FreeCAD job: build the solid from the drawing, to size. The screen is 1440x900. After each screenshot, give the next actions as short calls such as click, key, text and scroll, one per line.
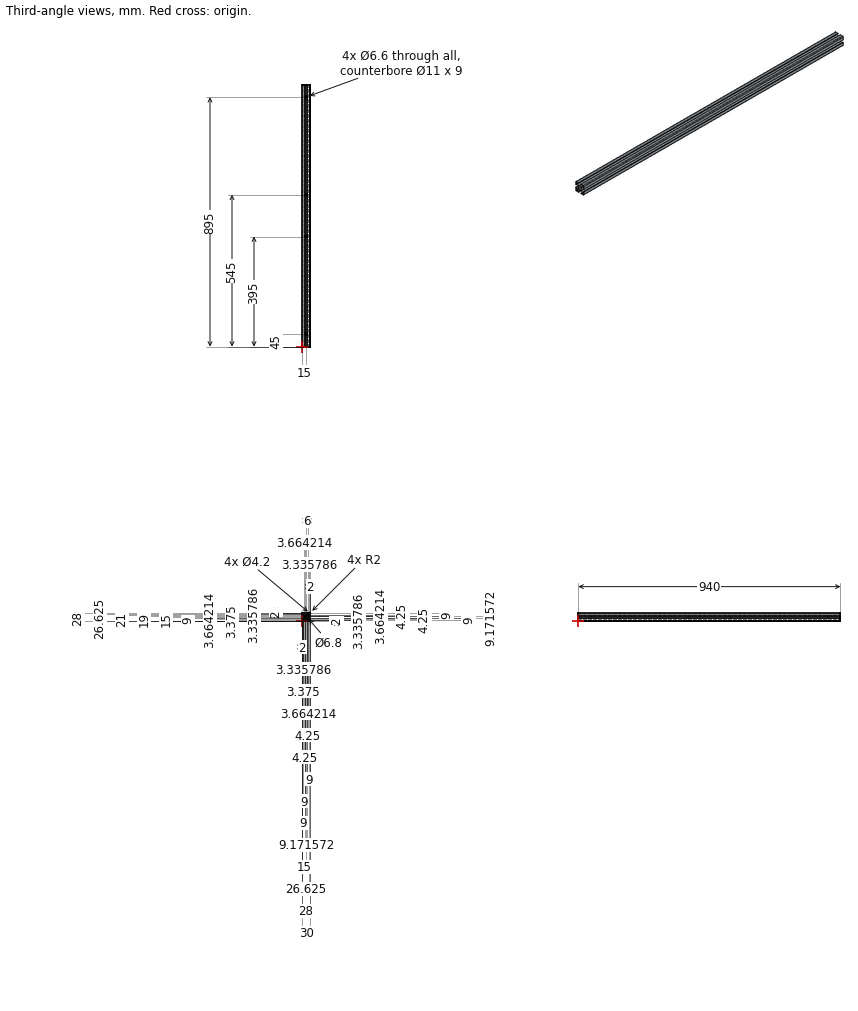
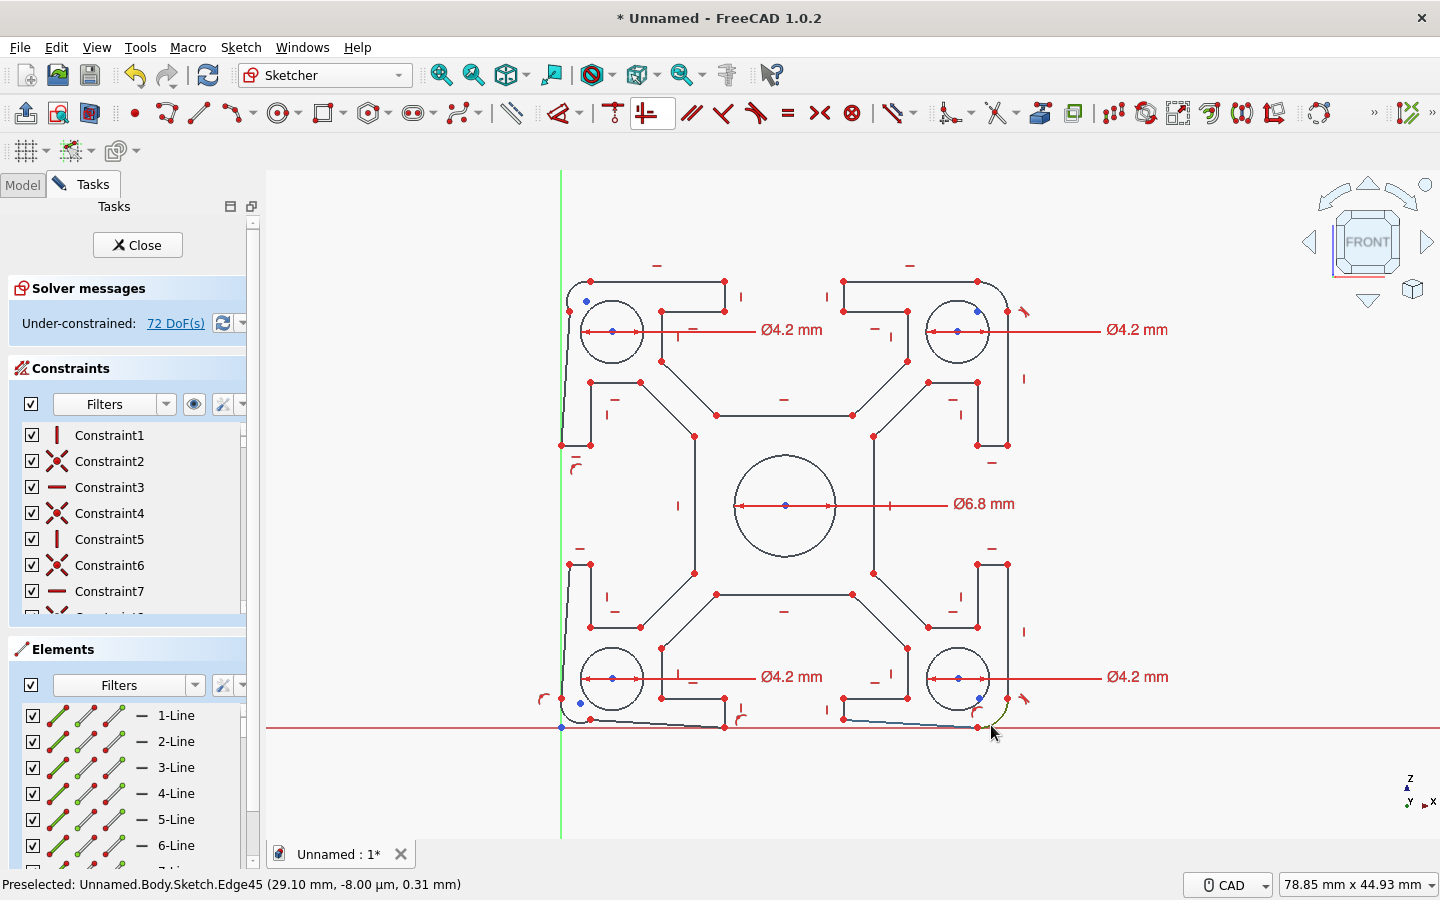
click(756, 114)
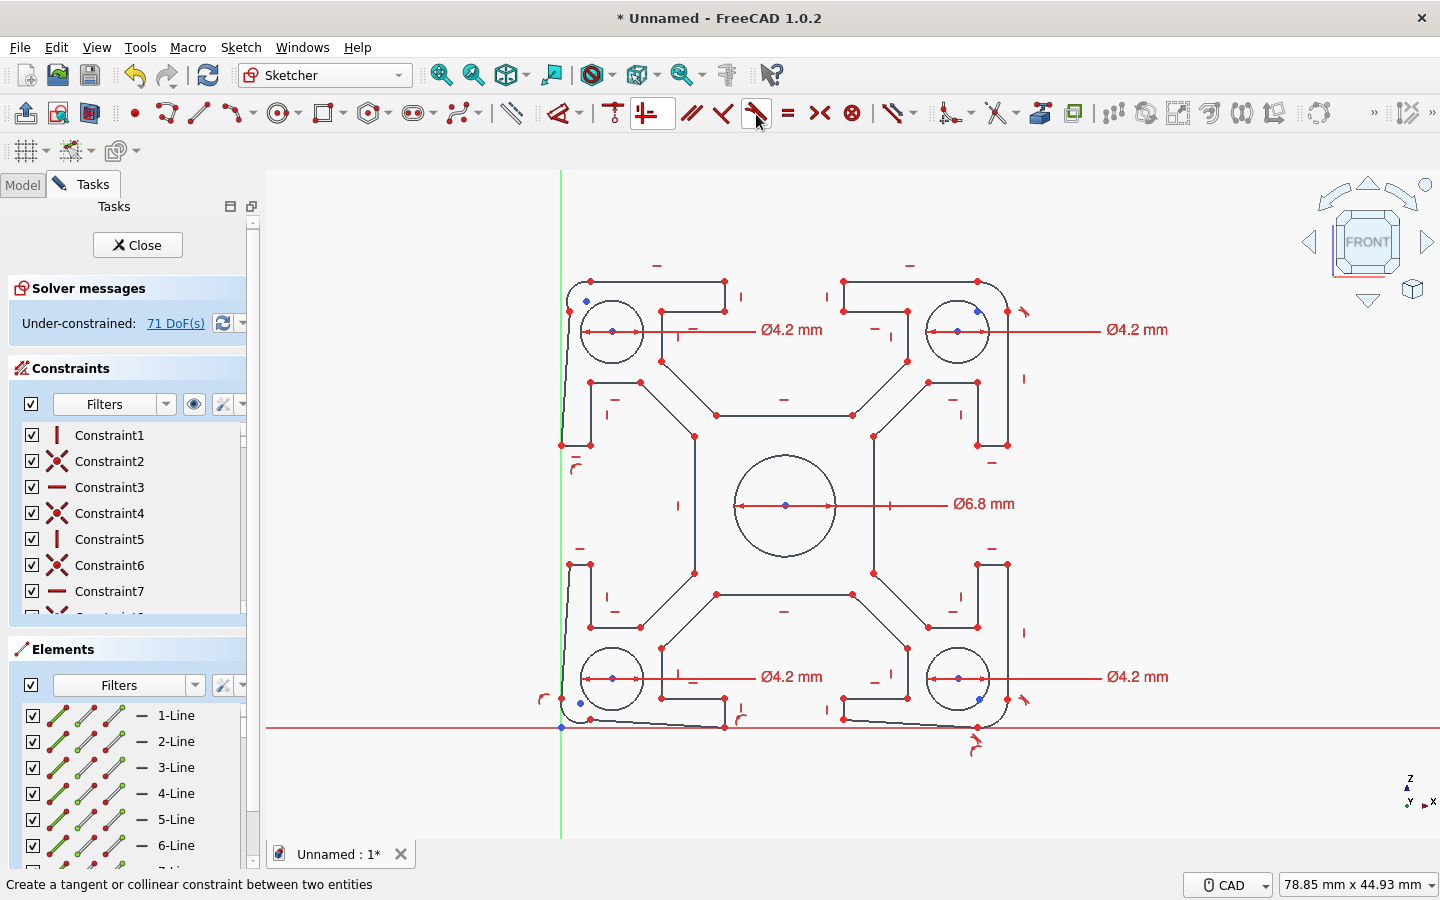
click(685, 726)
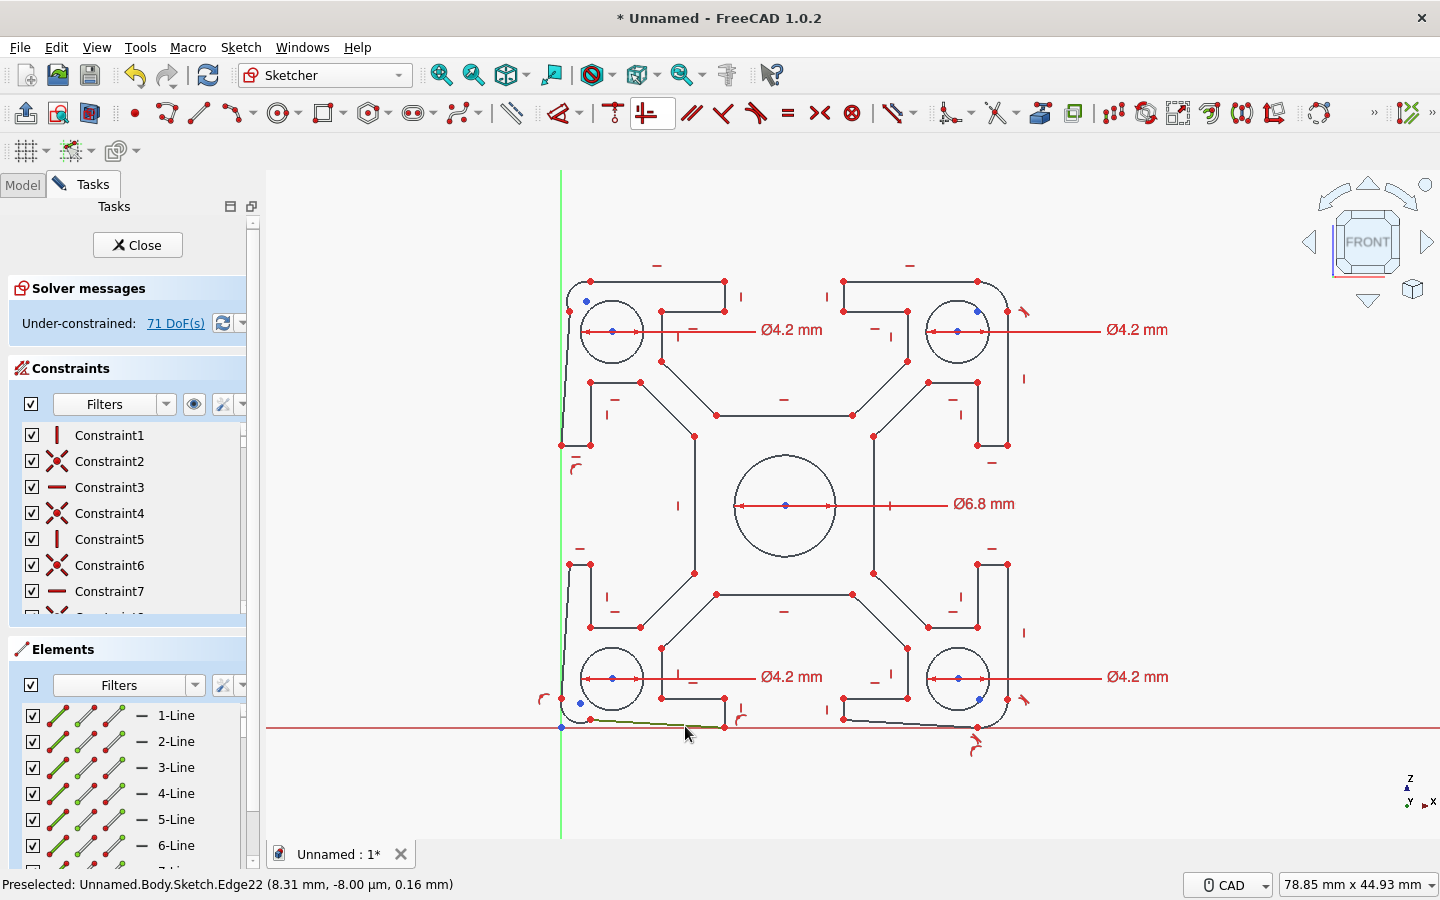
click(563, 712)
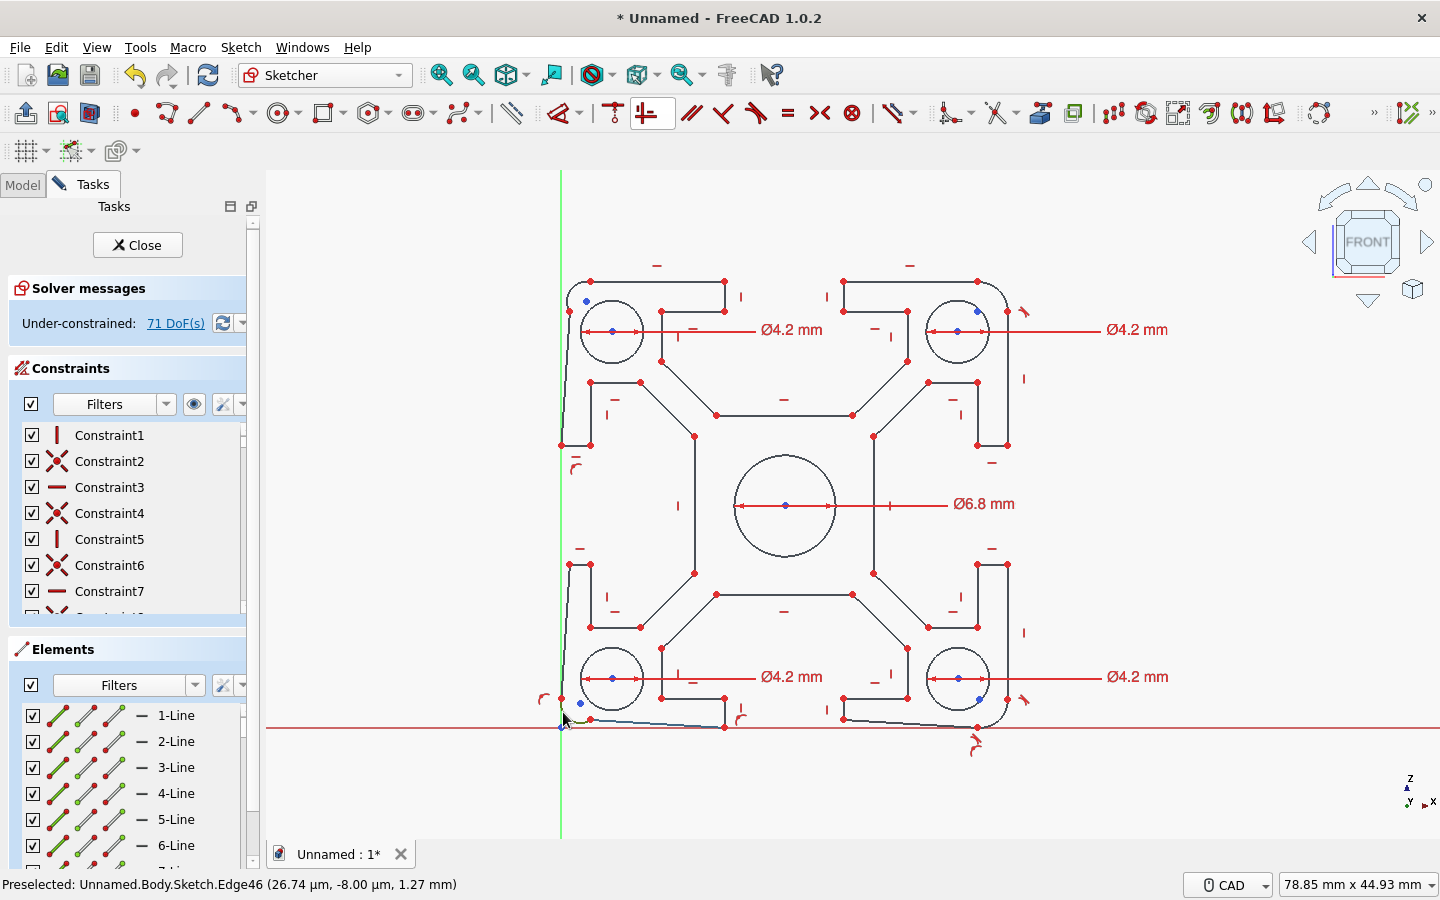
click(756, 114)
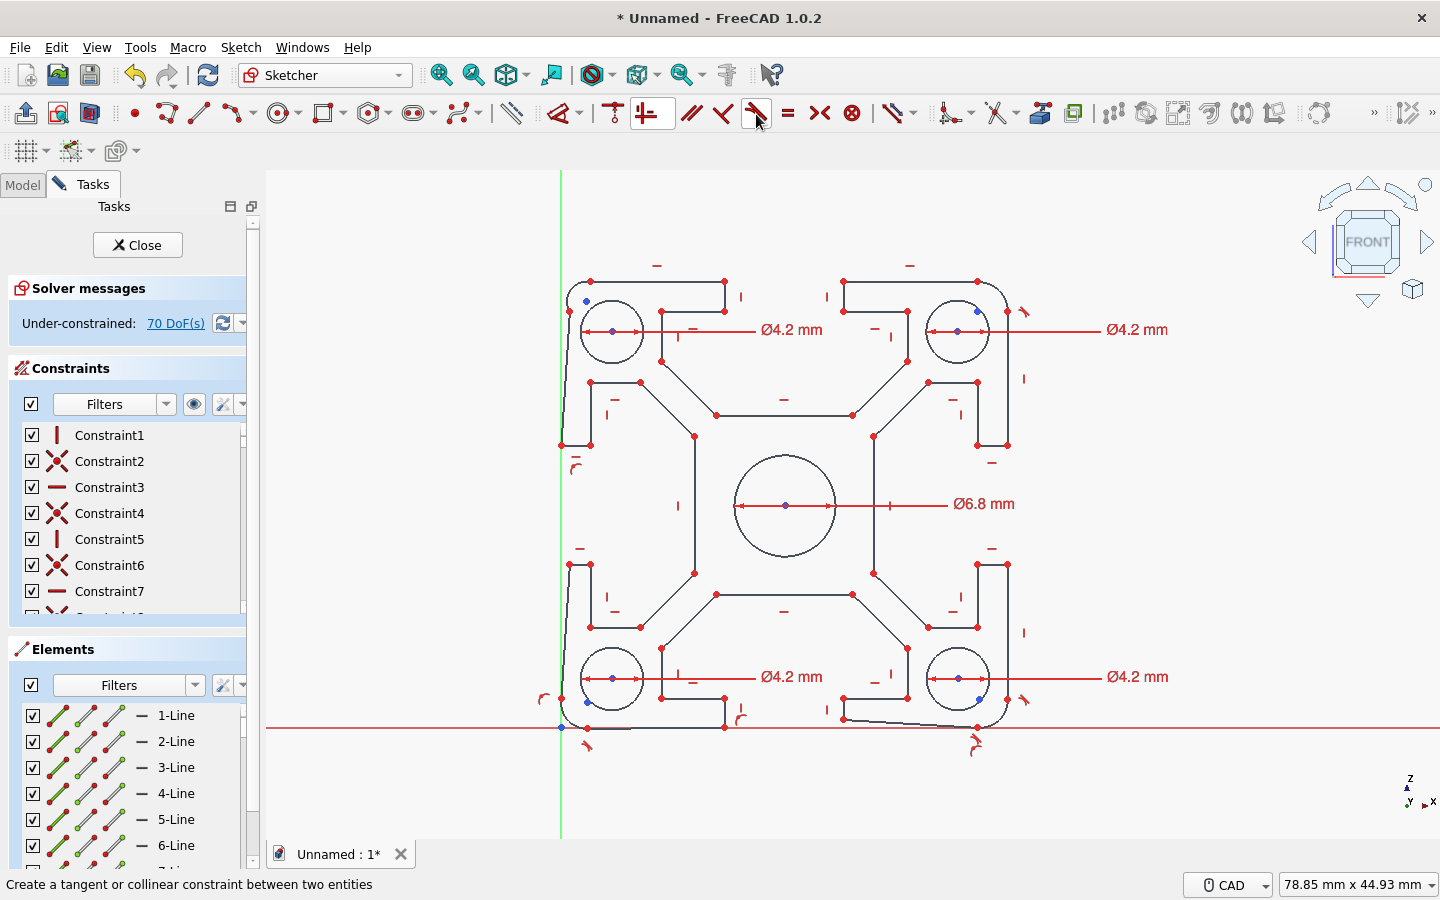
click(564, 659)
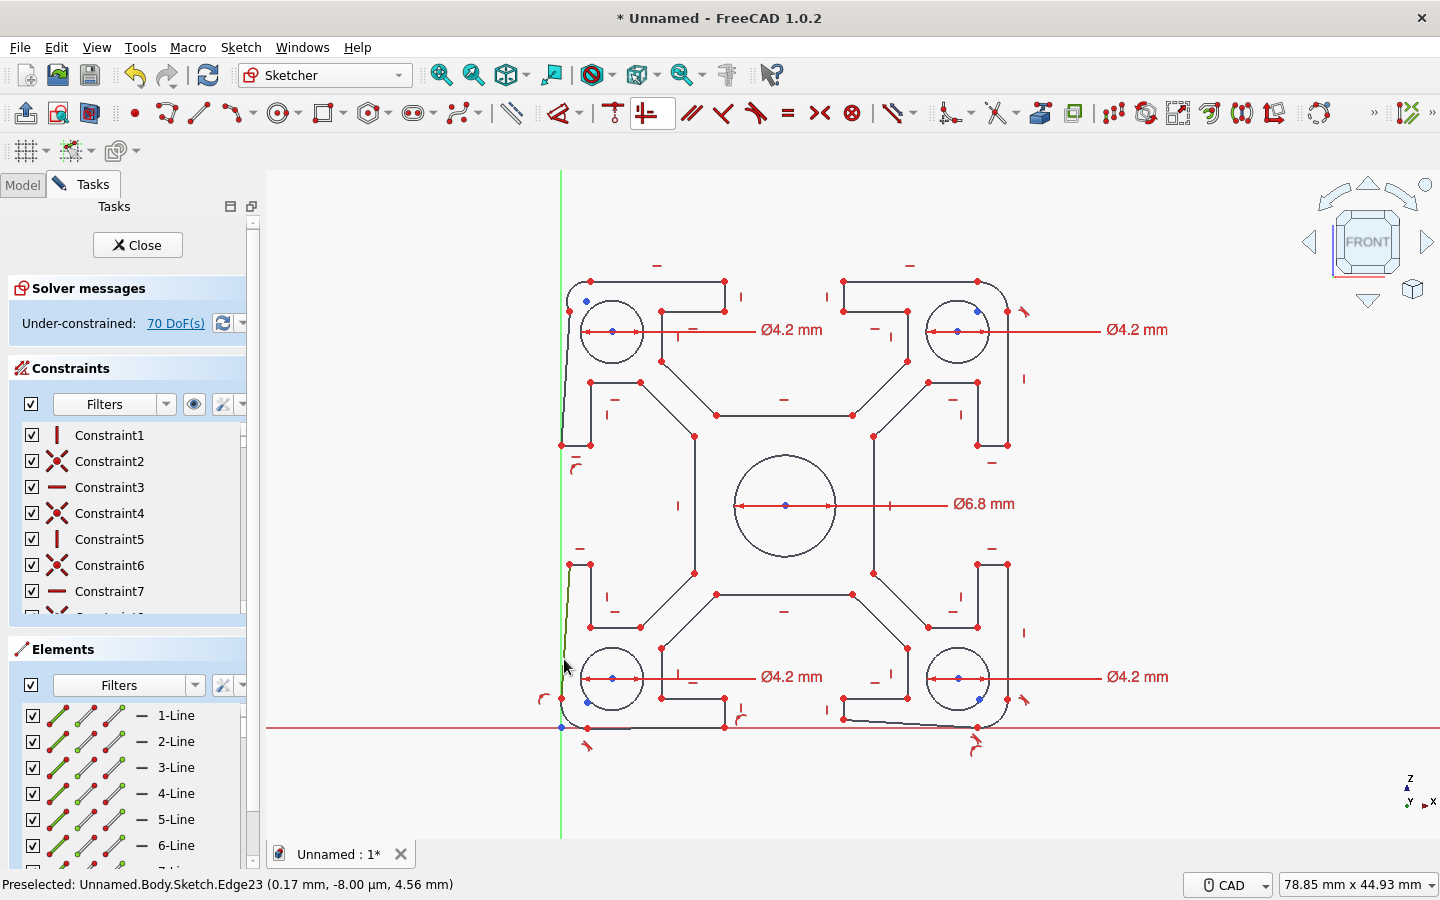
click(563, 712)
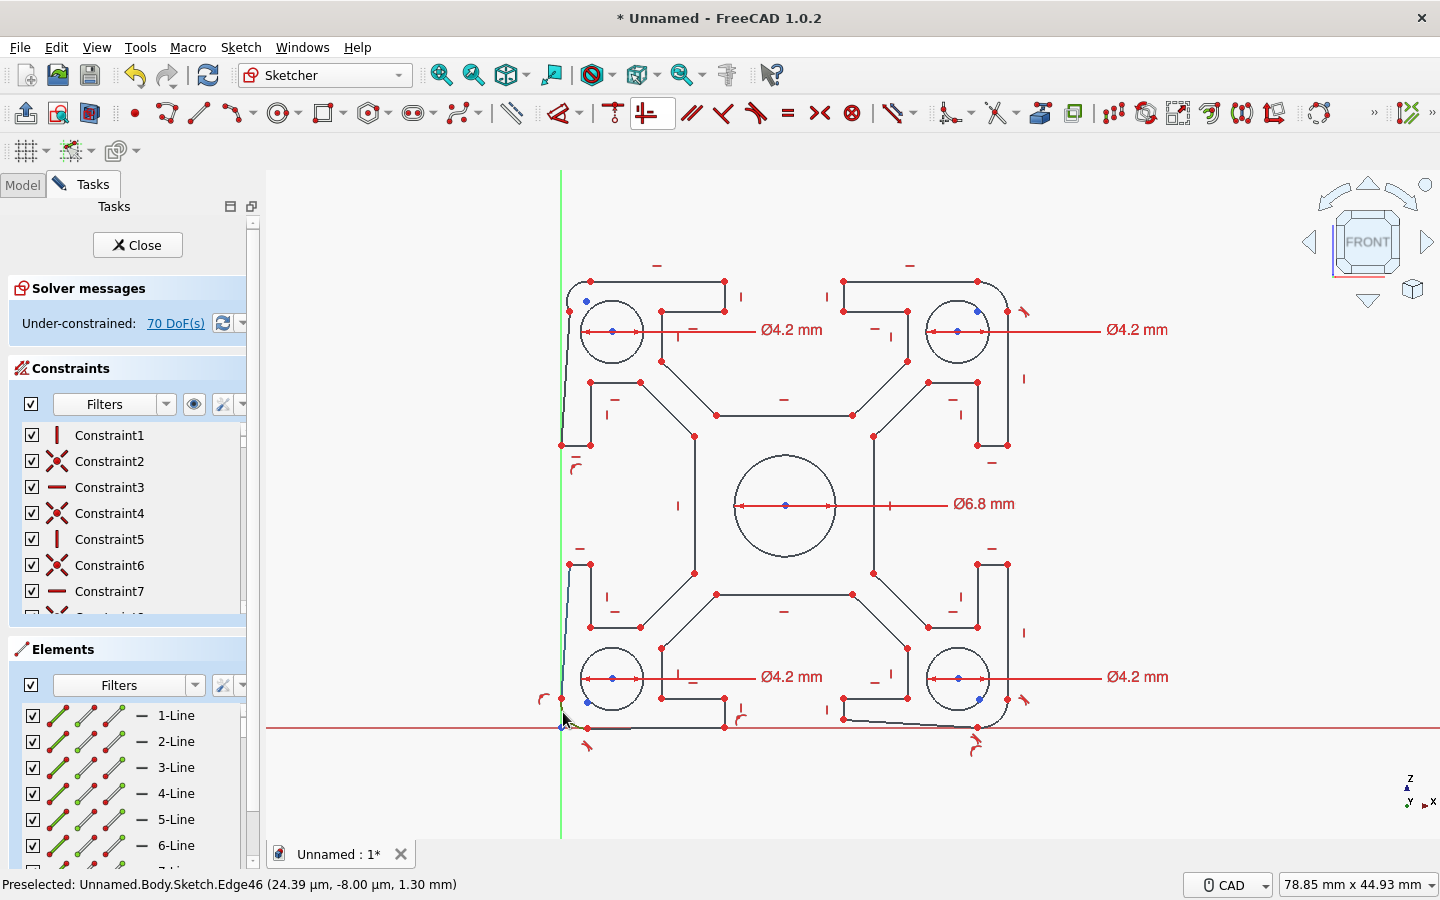
click(756, 114)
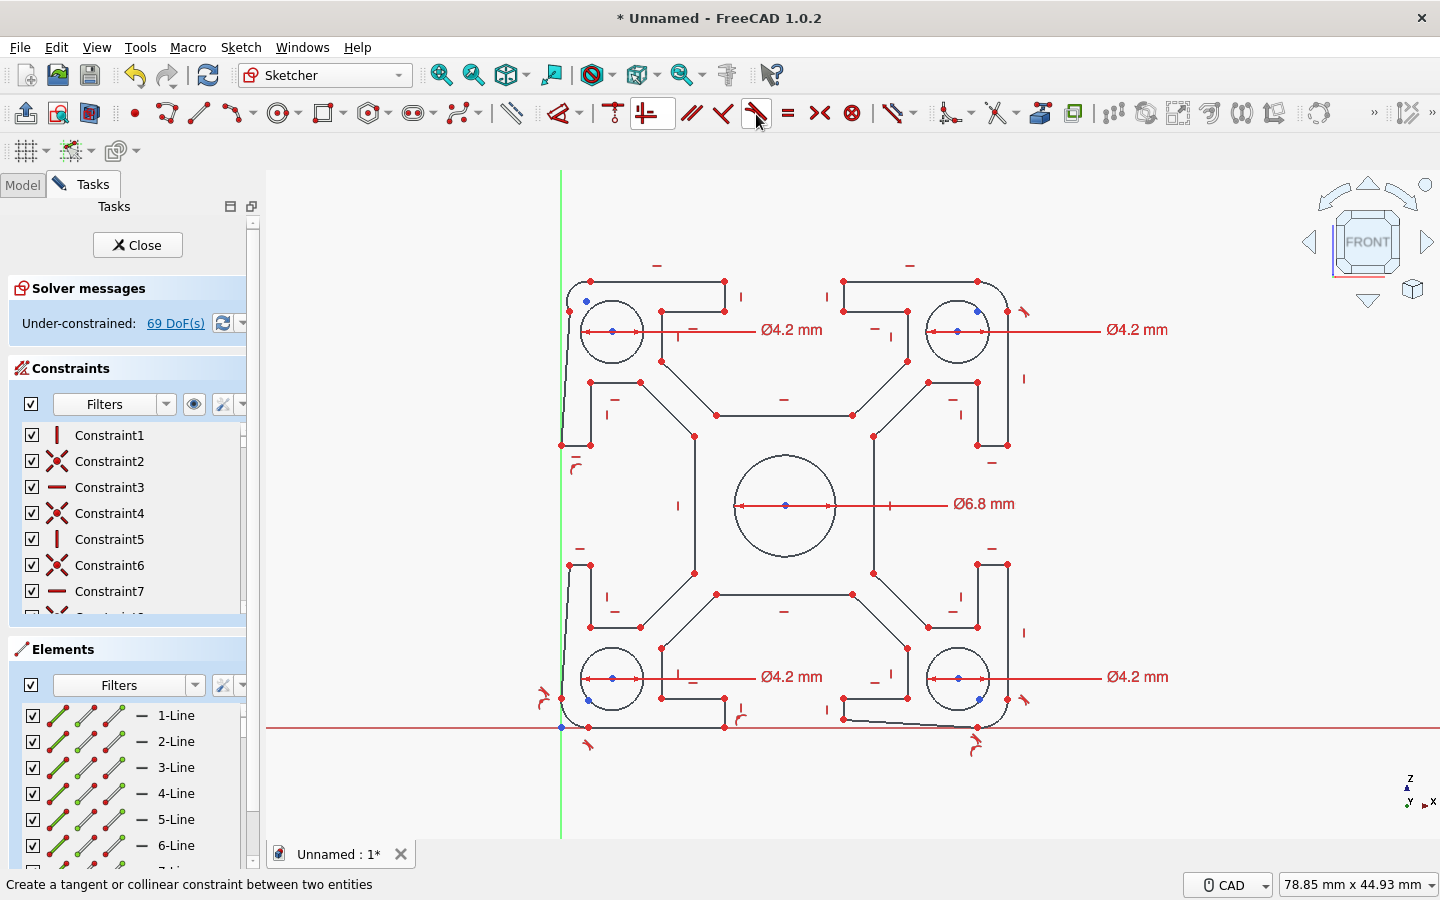
click(564, 406)